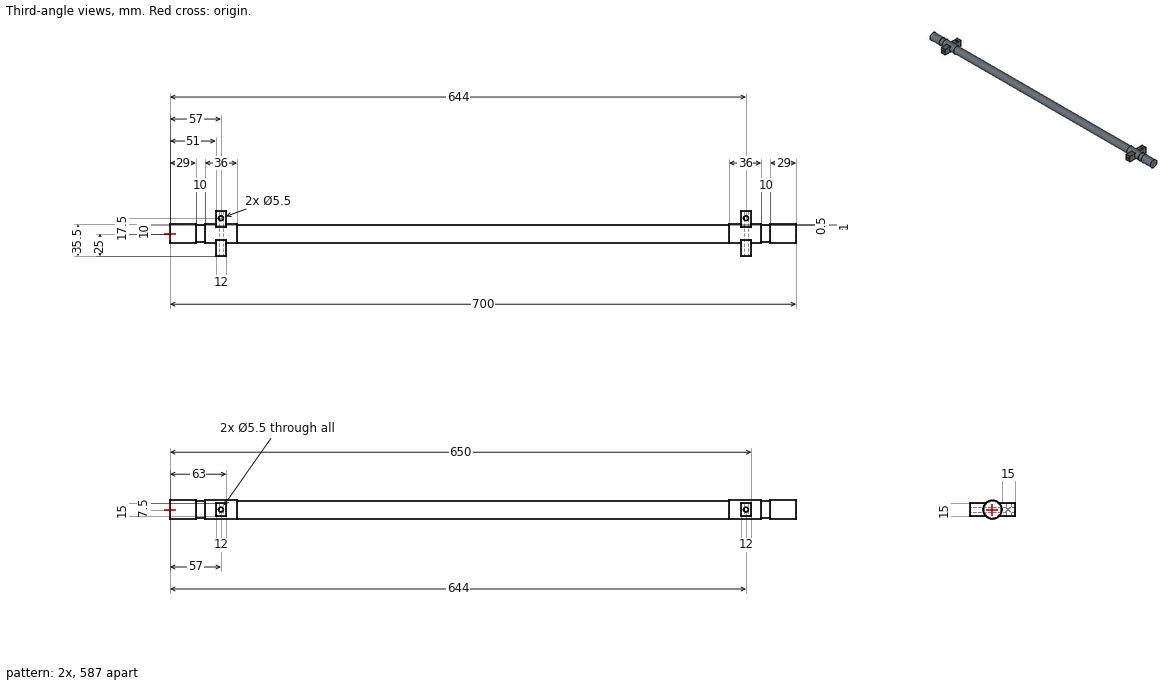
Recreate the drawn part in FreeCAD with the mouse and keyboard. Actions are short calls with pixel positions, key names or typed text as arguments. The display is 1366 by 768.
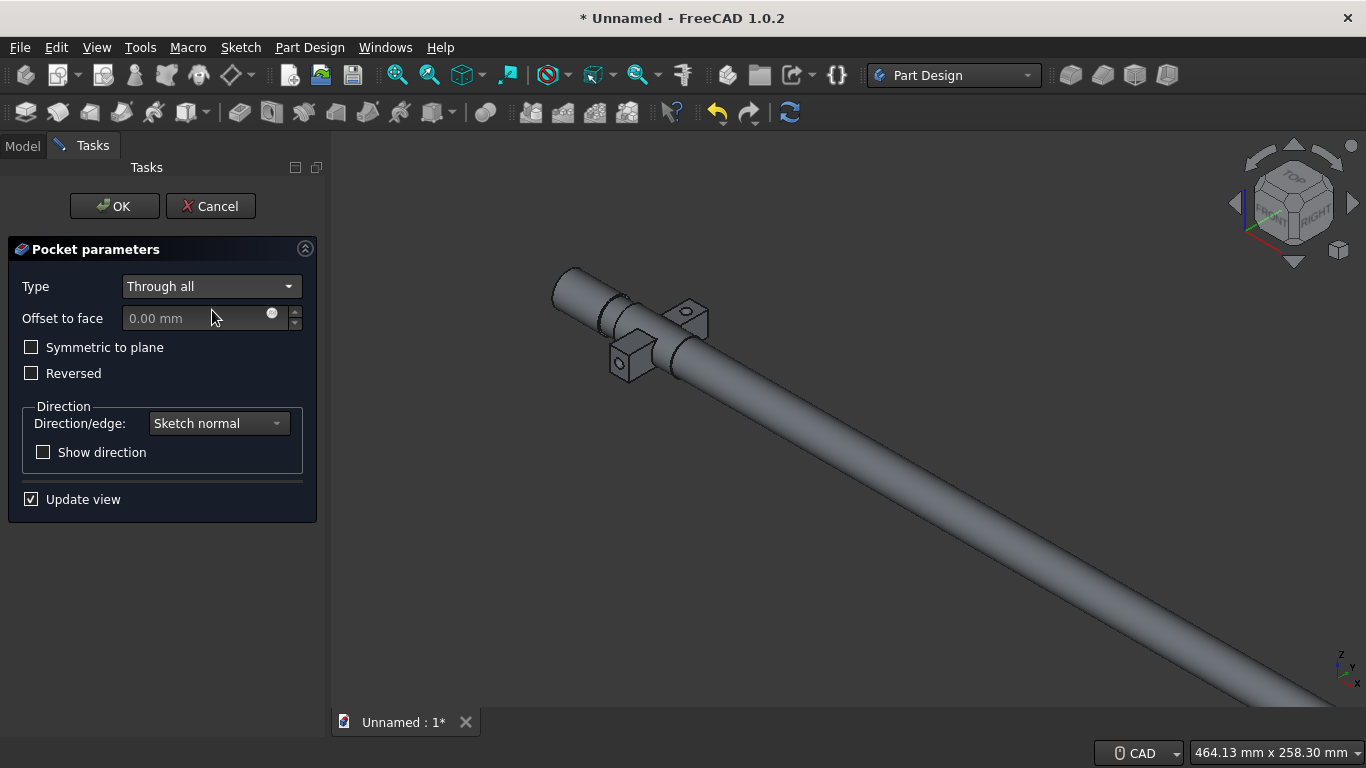
click(115, 206)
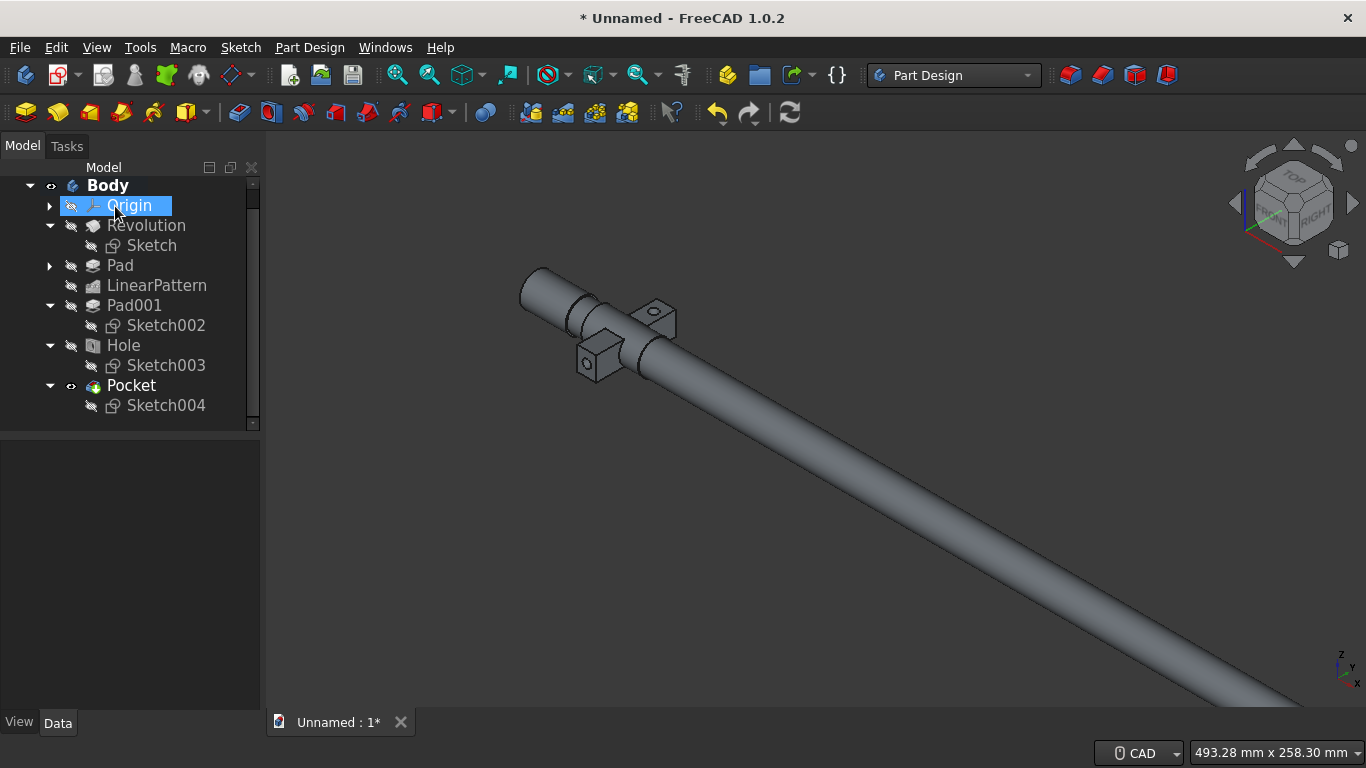
click(398, 76)